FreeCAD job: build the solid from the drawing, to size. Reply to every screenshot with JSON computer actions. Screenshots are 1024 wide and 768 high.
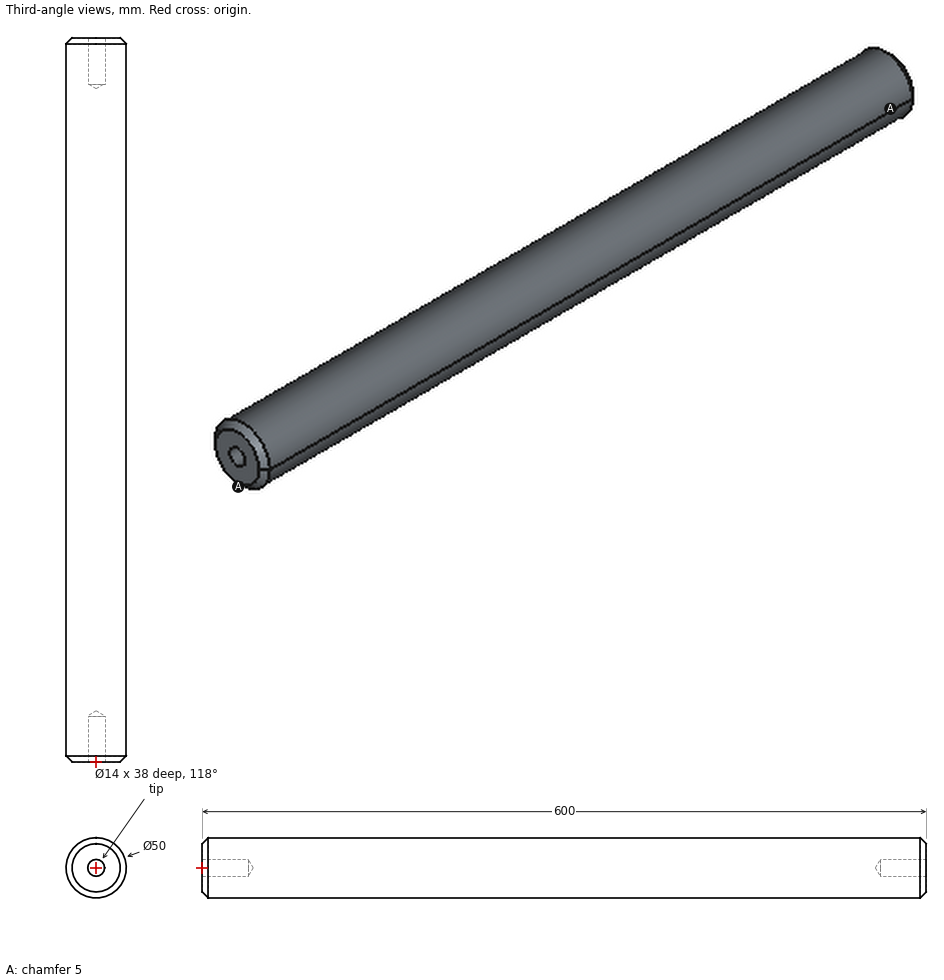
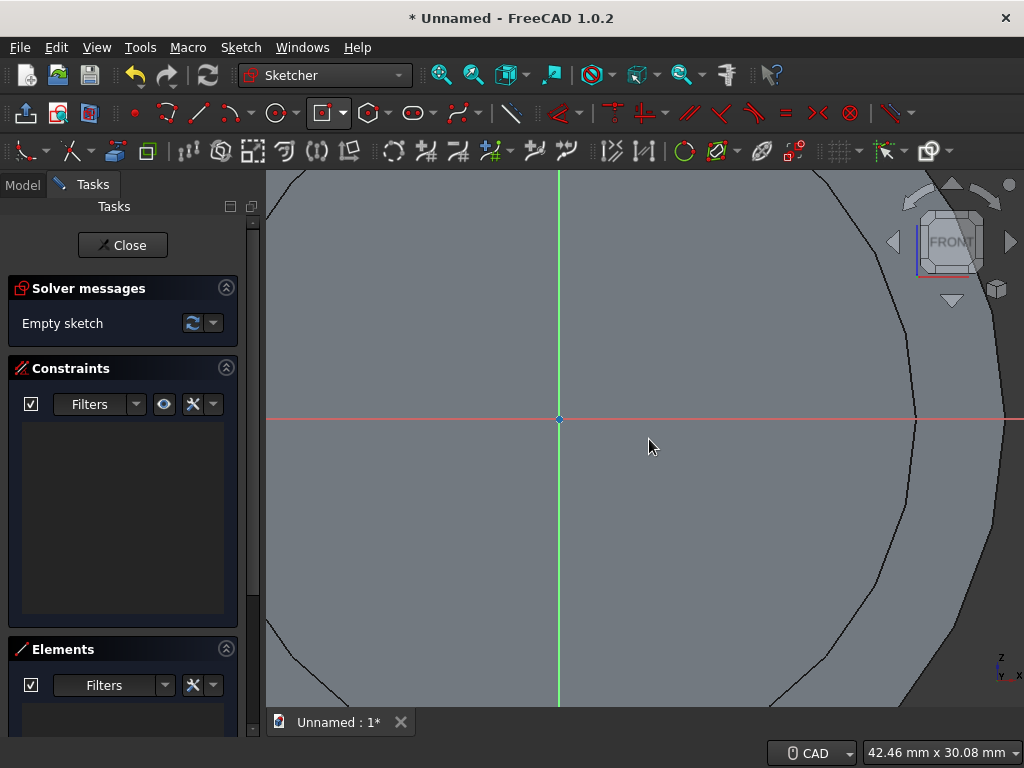
{"action": "scroll", "coordinate": [523, 381], "scroll_direction": "up", "scroll_amount": 2}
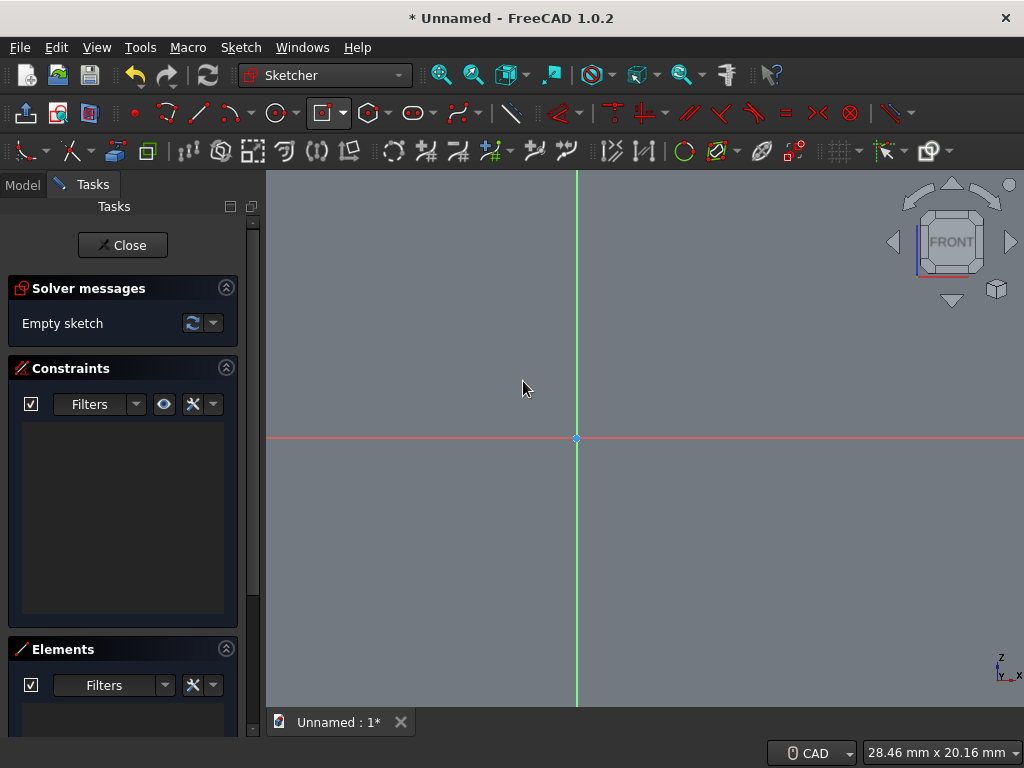
{"action": "left_click", "coordinate": [276, 114]}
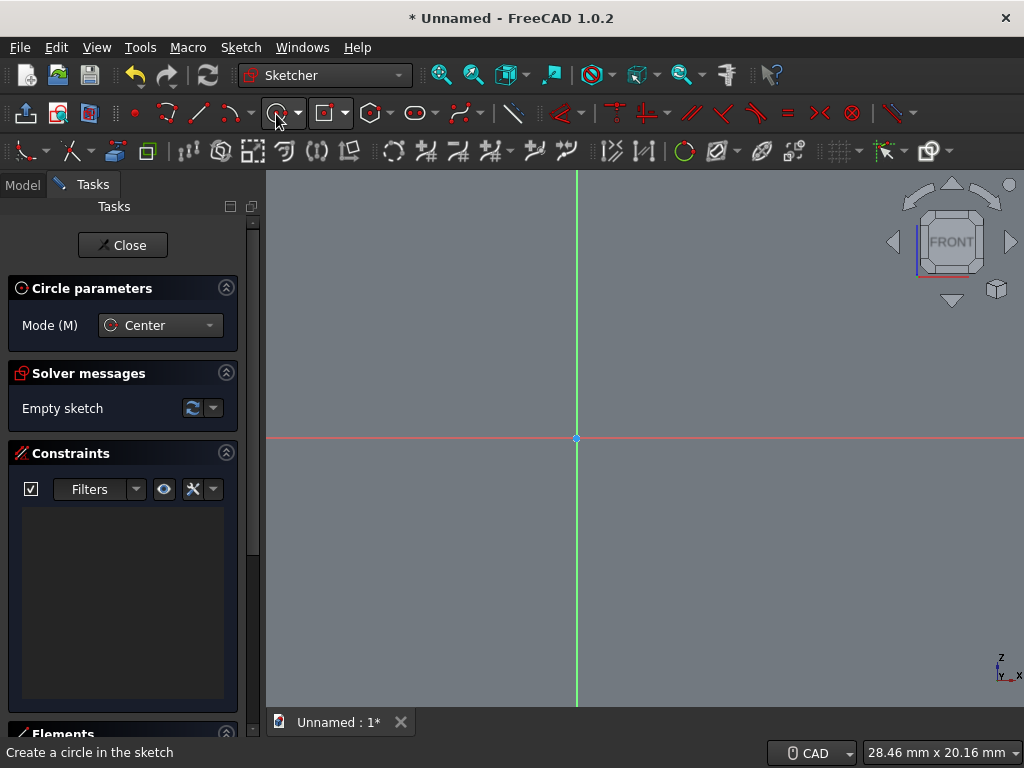
{"action": "left_click", "coordinate": [577, 438]}
{"action": "mouse_move", "coordinate": [708, 306]}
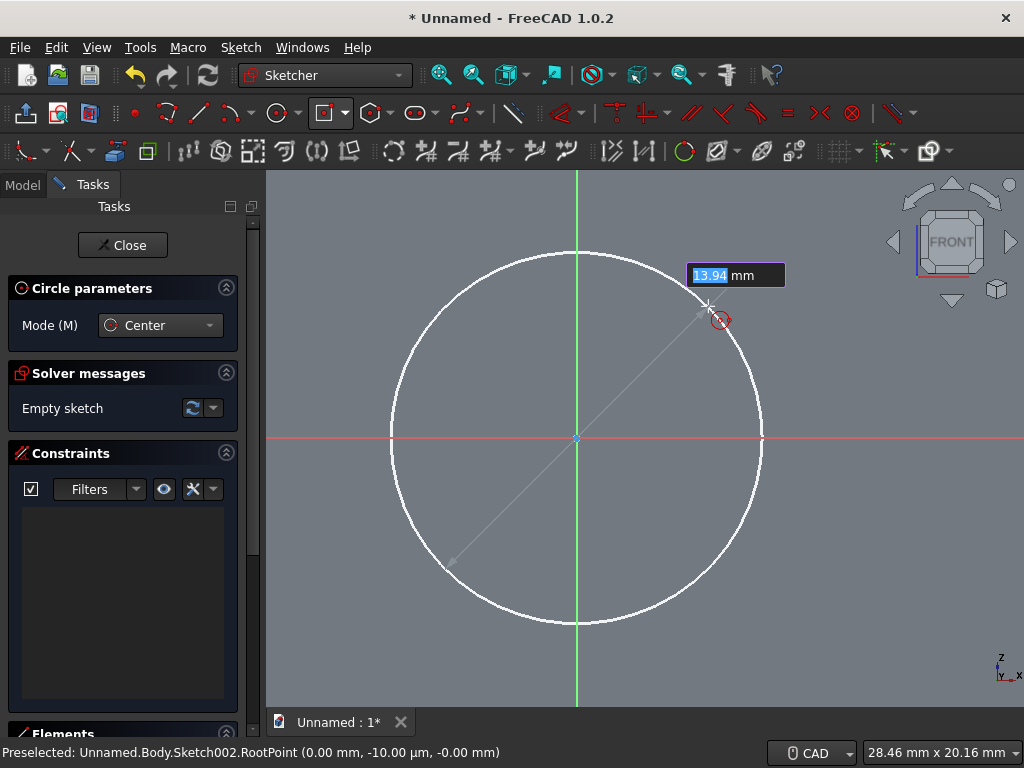
{"action": "type", "text": "14"}
{"action": "key", "text": "Return"}
{"action": "key", "text": "Escape"}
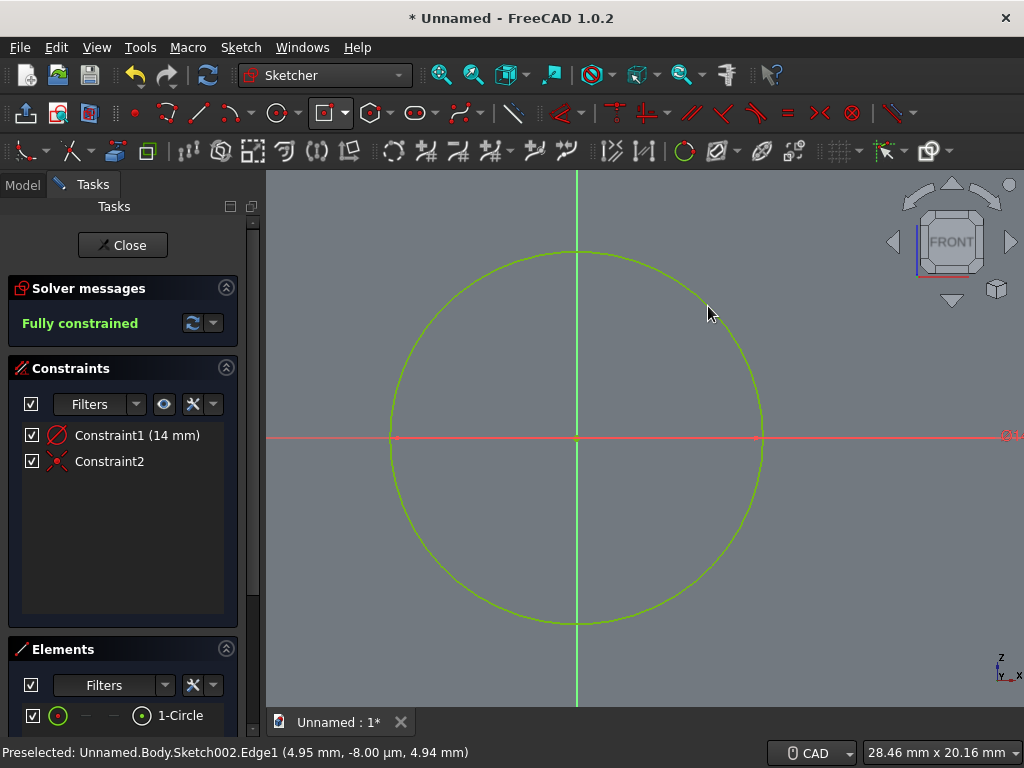
{"action": "left_click", "coordinate": [123, 245]}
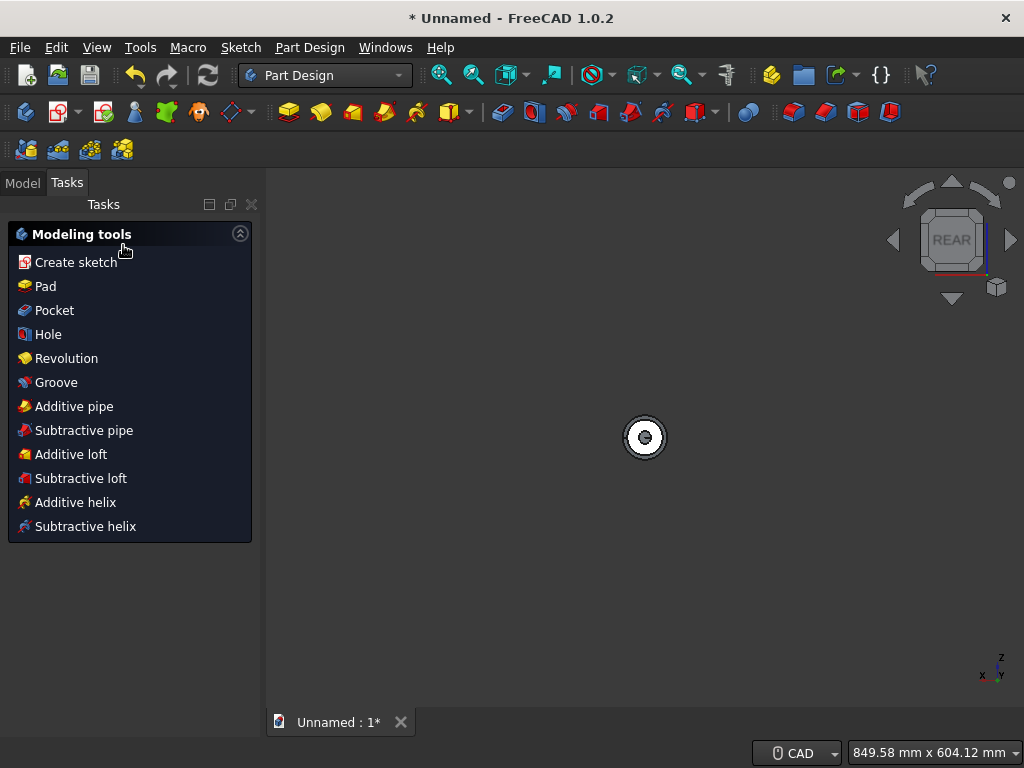
{"action": "left_click", "coordinate": [536, 112]}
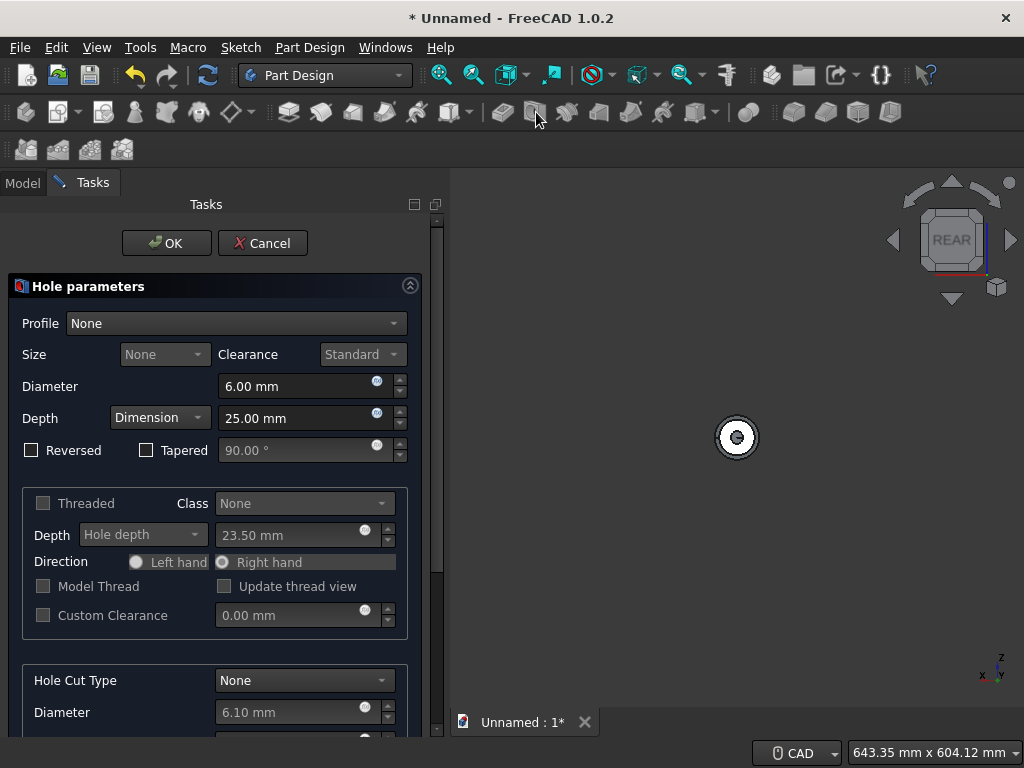
{"action": "triple_click", "coordinate": [305, 386]}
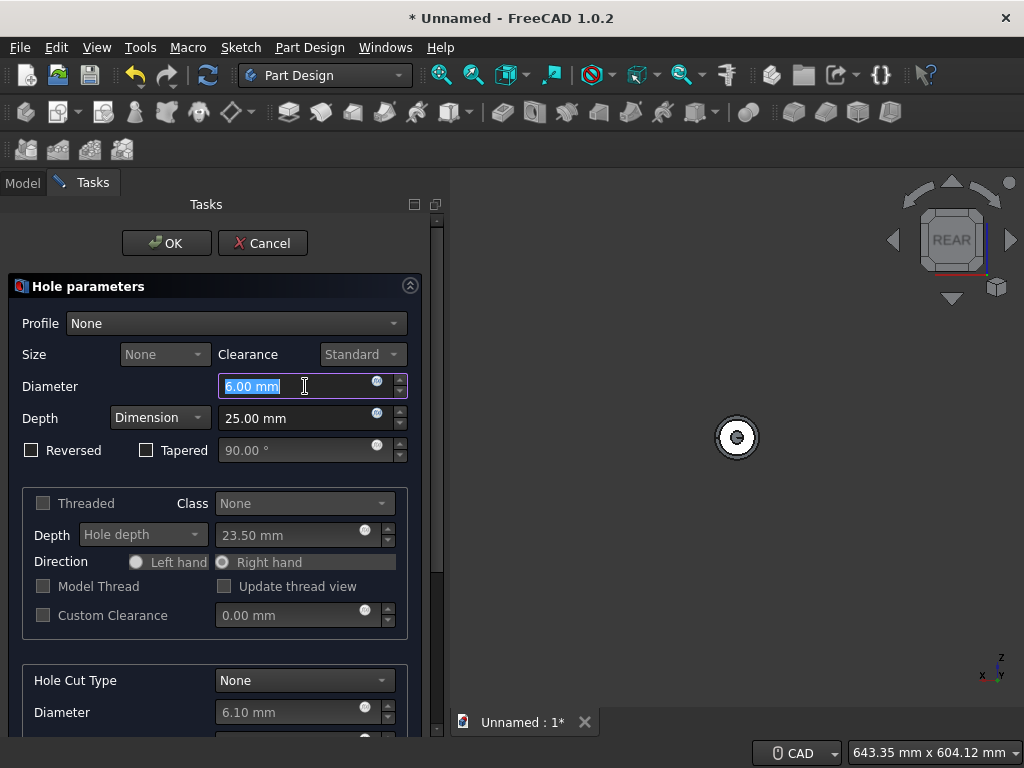
{"action": "type", "text": "14"}
{"action": "key", "text": "Tab"}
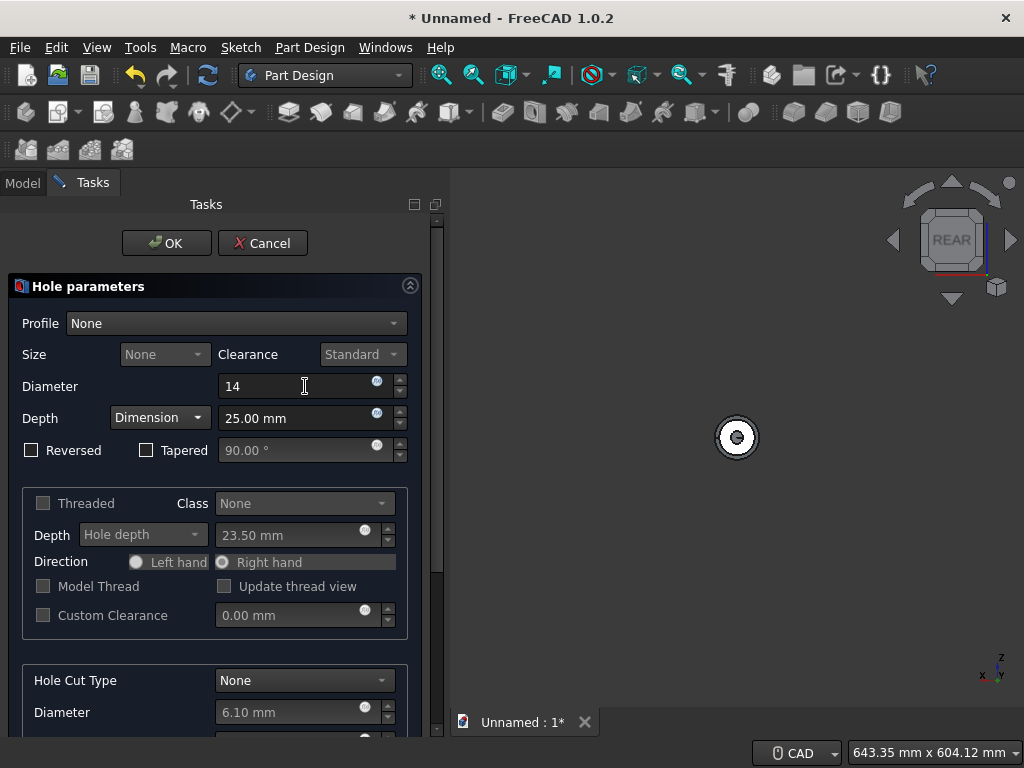
{"action": "triple_click", "coordinate": [305, 418]}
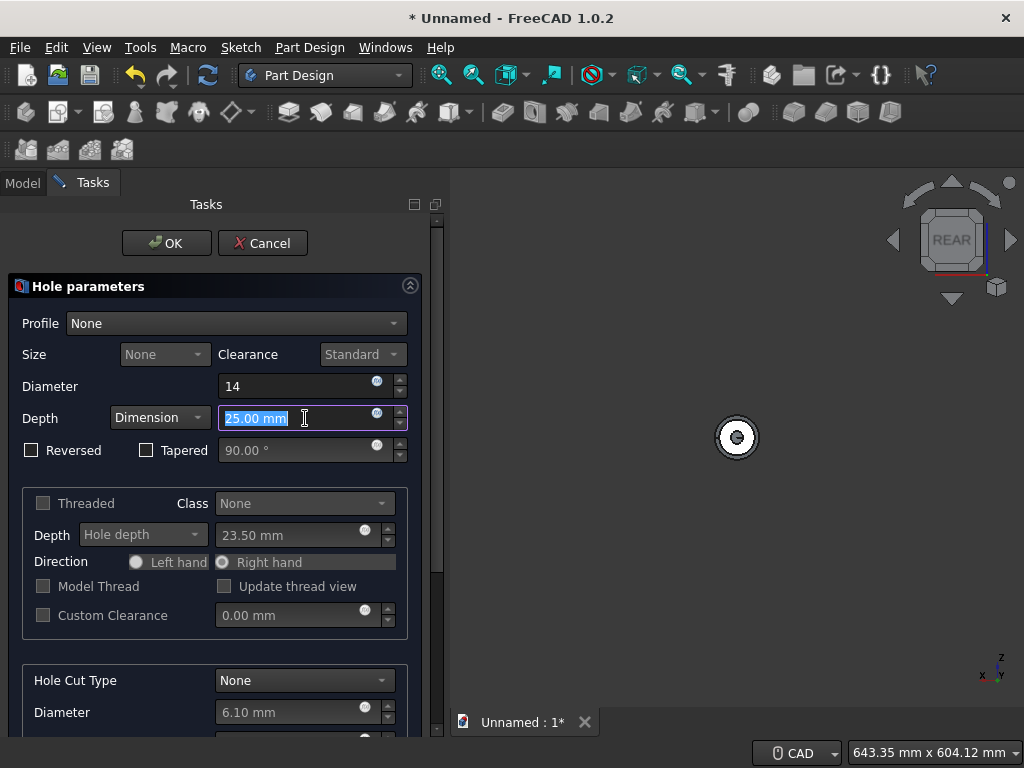
{"action": "type", "text": "38"}
{"action": "key", "text": "Tab"}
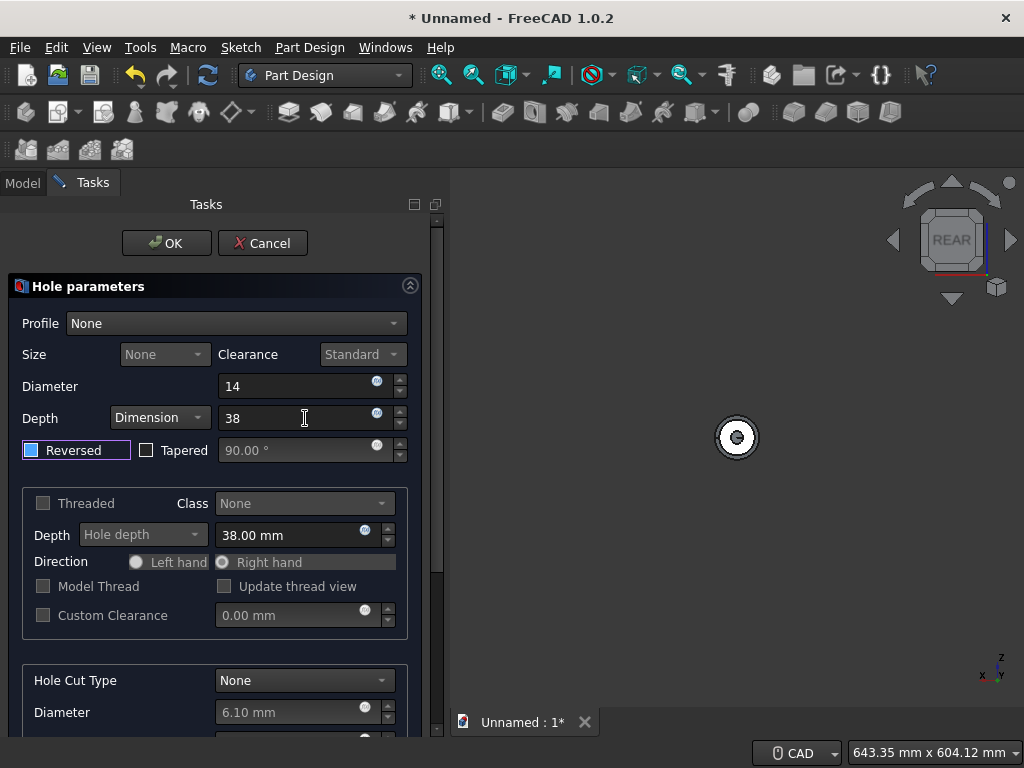
{"action": "left_click", "coordinate": [167, 243]}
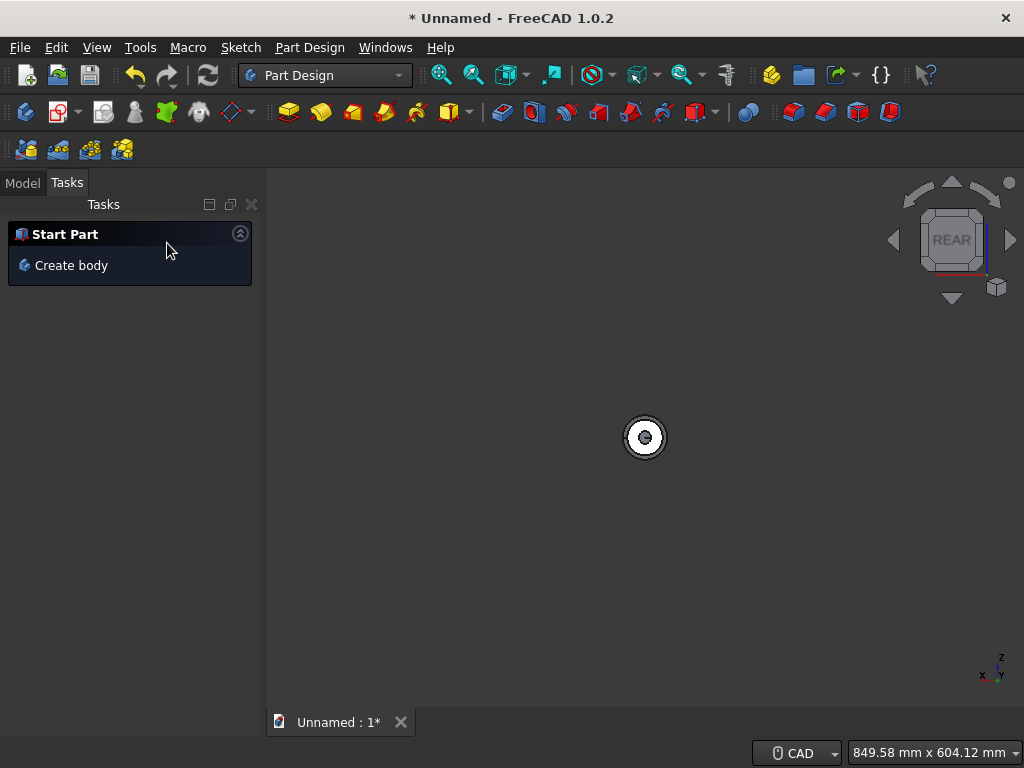
{"action": "key", "text": "0"}